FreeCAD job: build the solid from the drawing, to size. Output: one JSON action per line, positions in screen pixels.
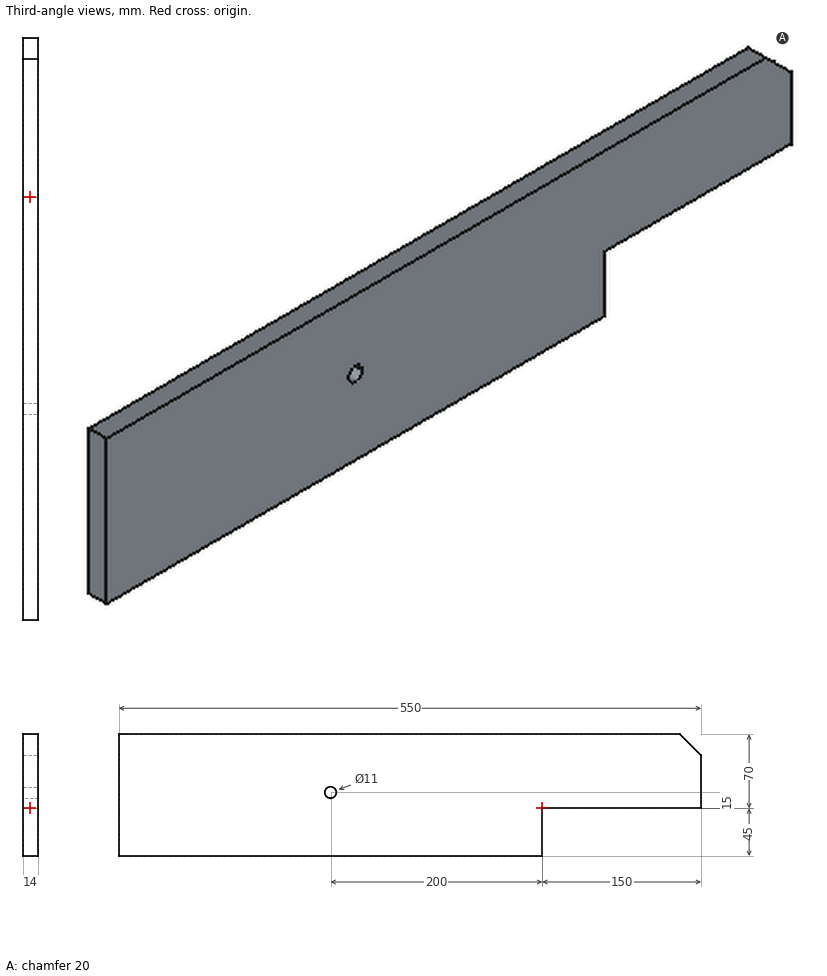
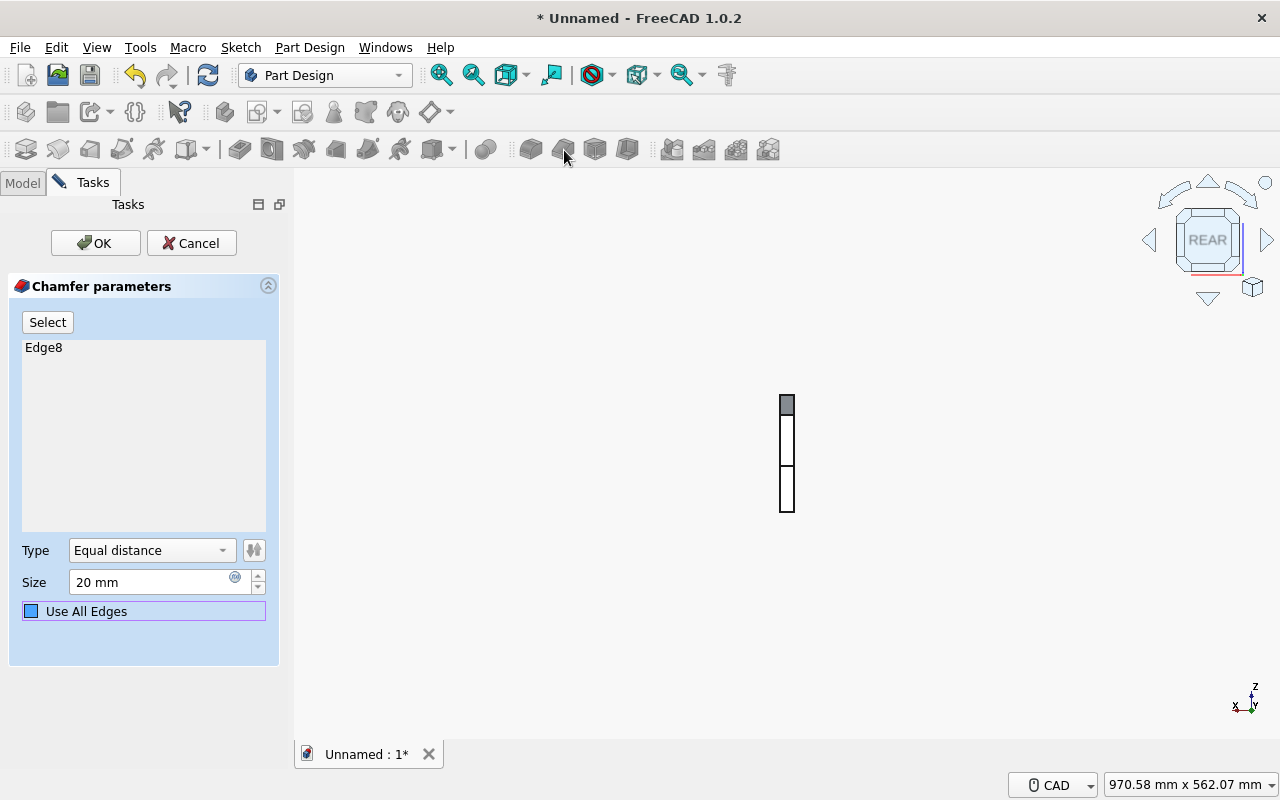
{"action": "left_click", "coordinate": [96, 243]}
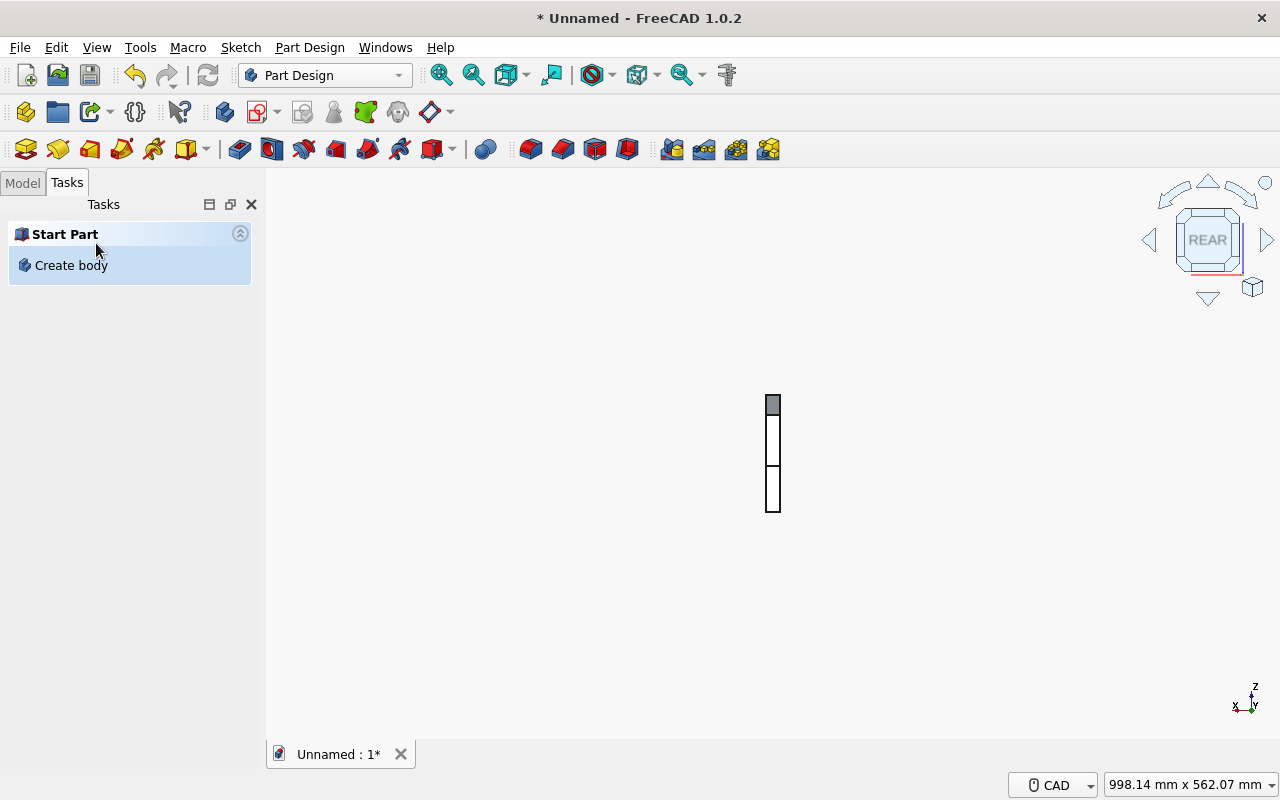
{"action": "key", "text": "0"}